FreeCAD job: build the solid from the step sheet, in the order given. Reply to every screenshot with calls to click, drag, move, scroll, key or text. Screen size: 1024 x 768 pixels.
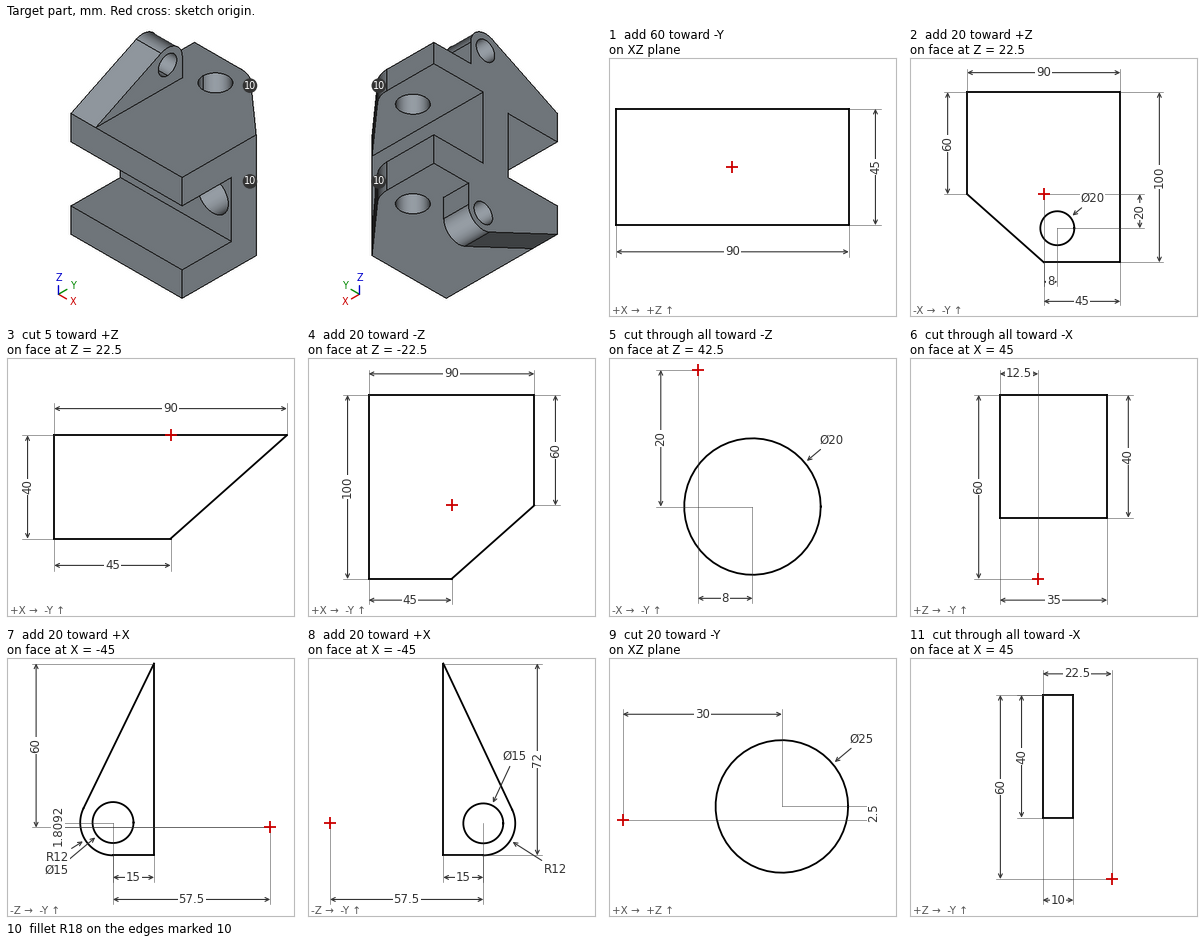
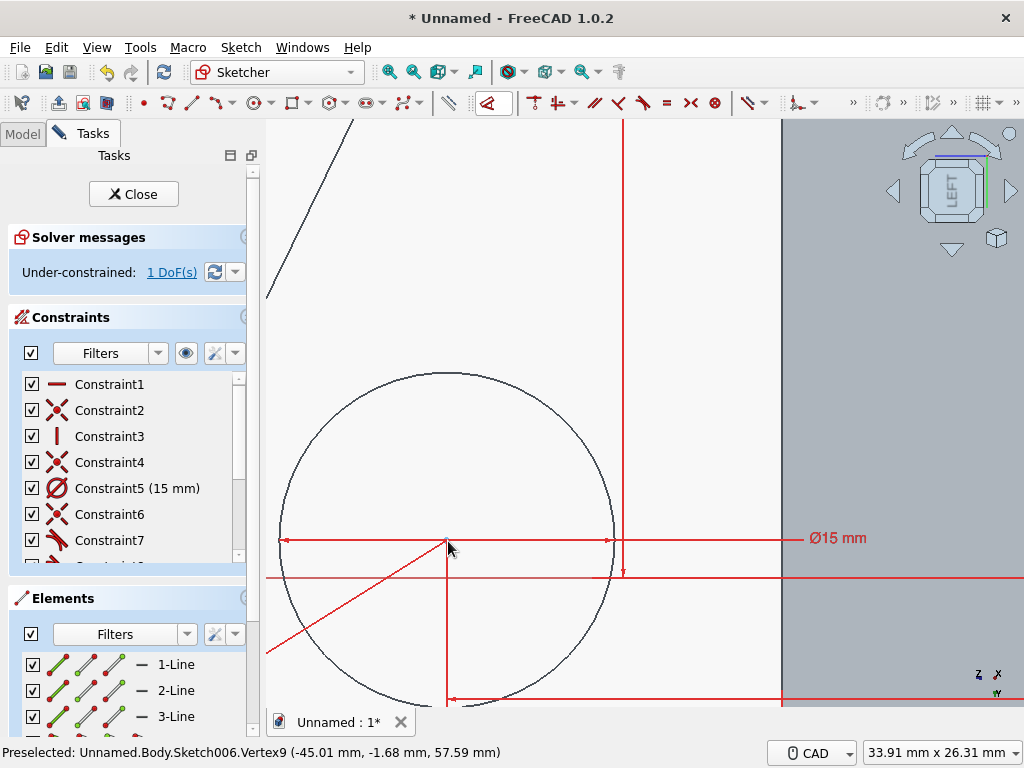
click(447, 540)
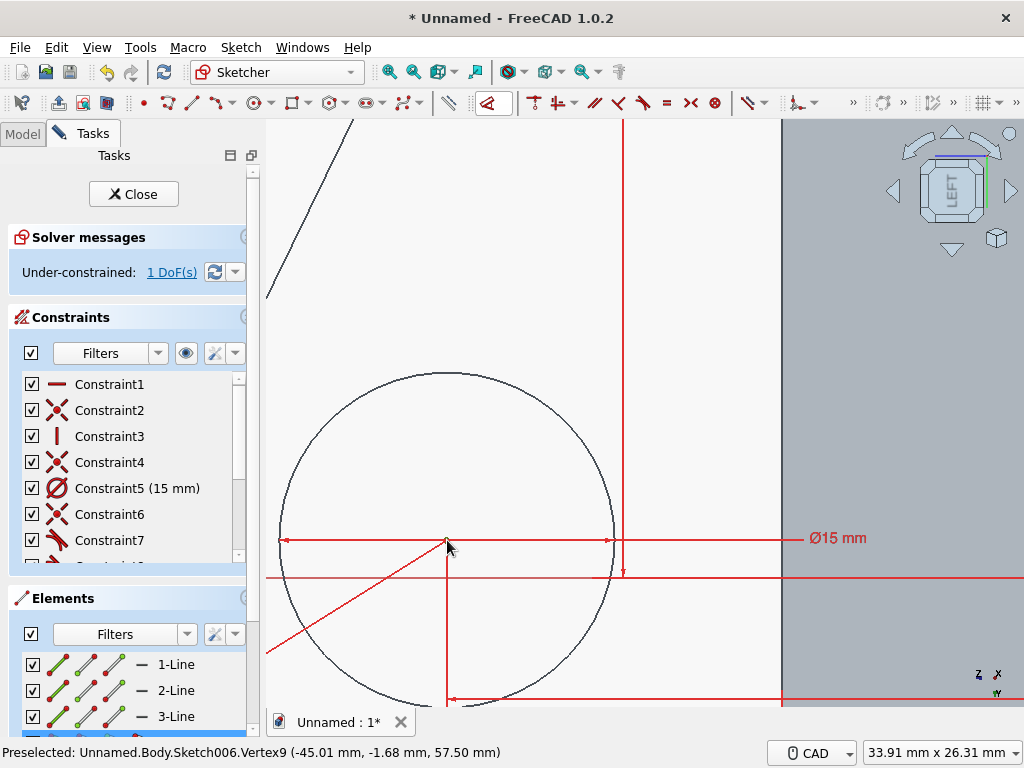
key(i)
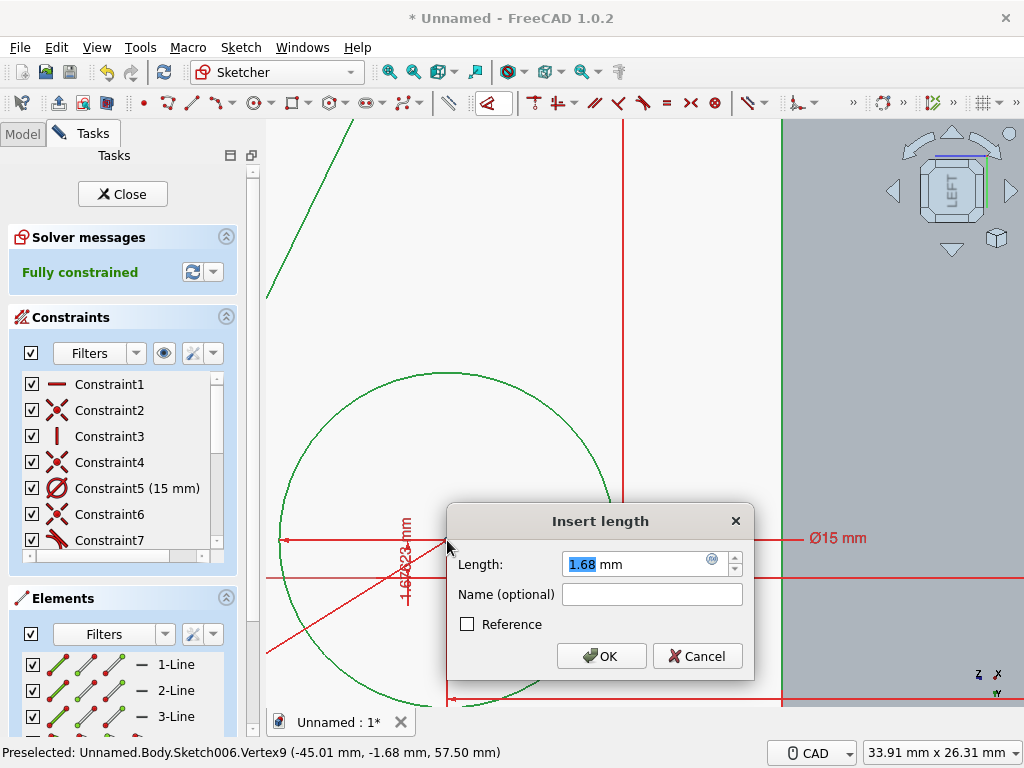
text(1.8092)
key(Return)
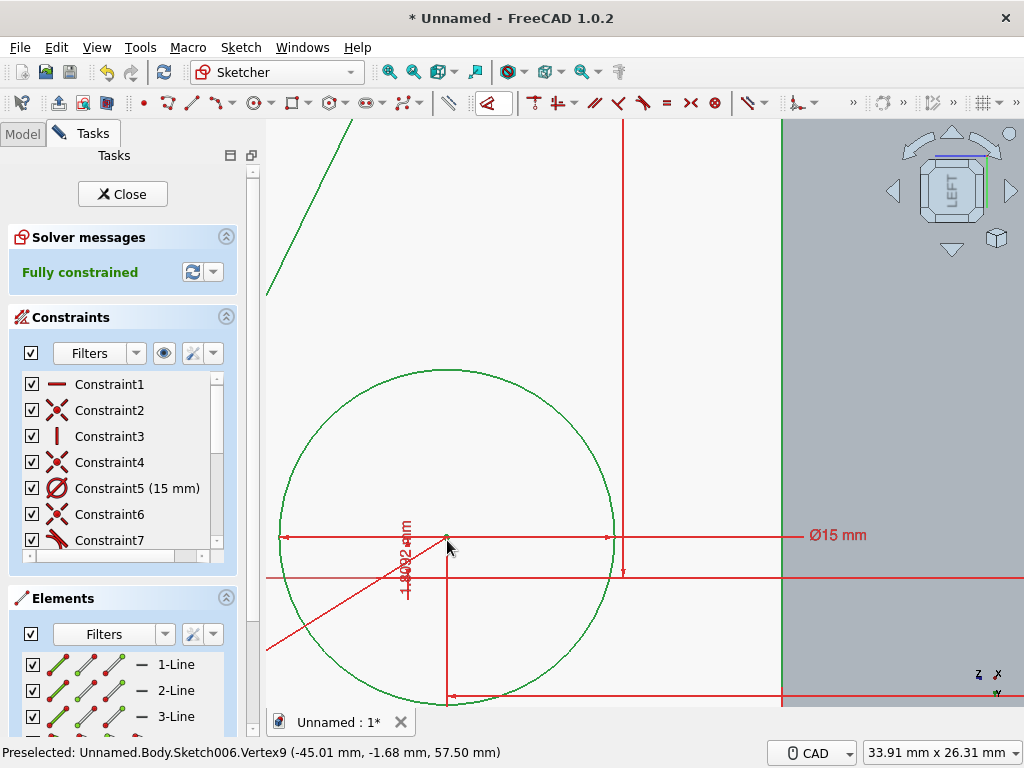
click(123, 194)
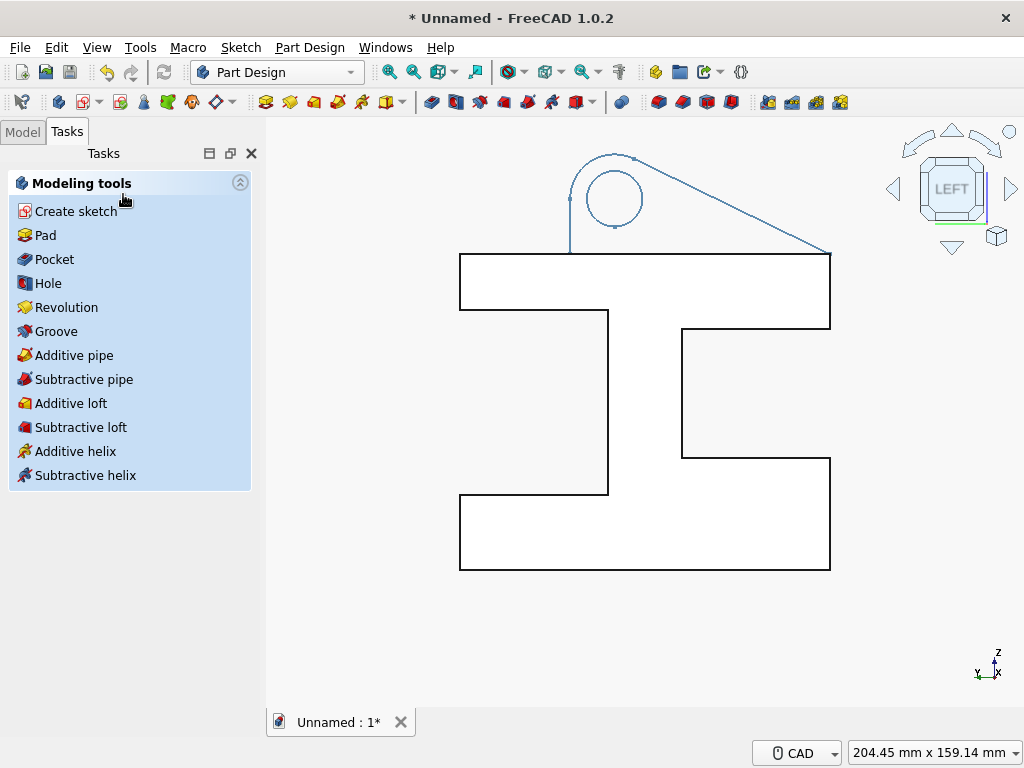
click(266, 102)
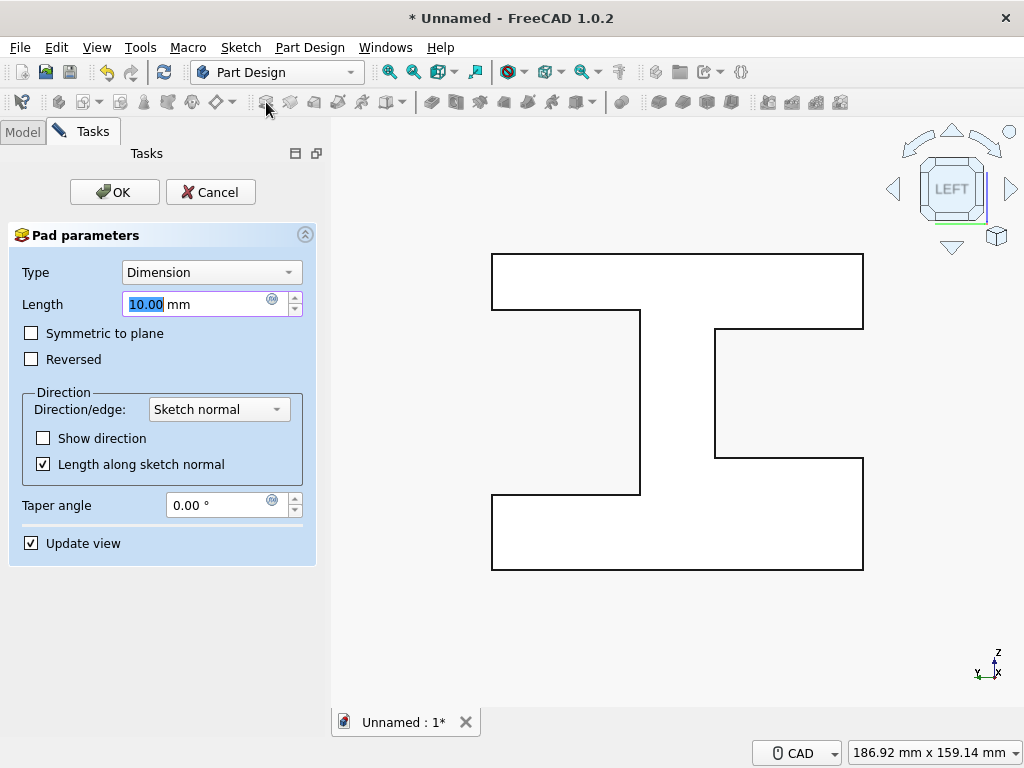
text(20)
key(Tab)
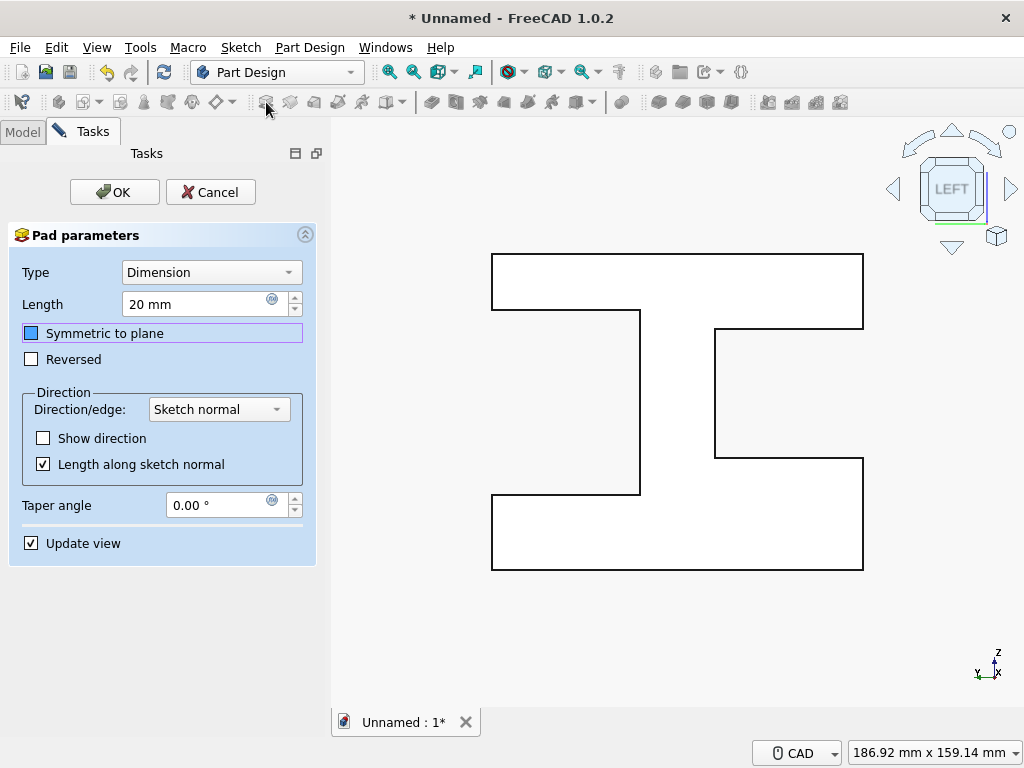
click(30, 359)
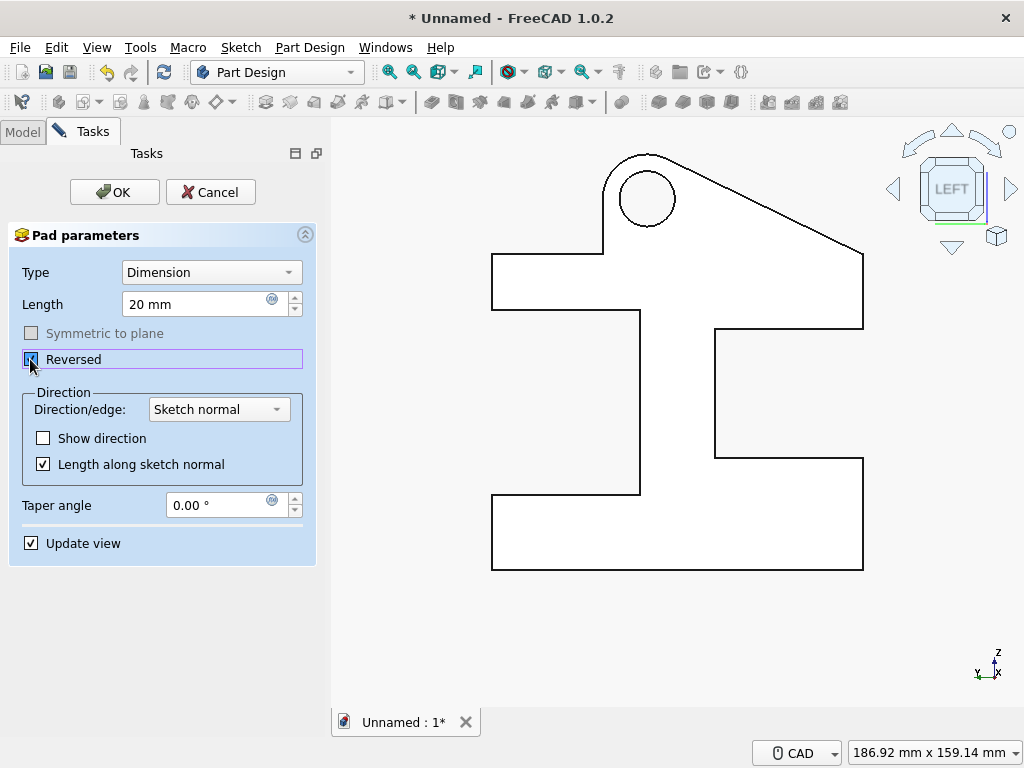
click(115, 192)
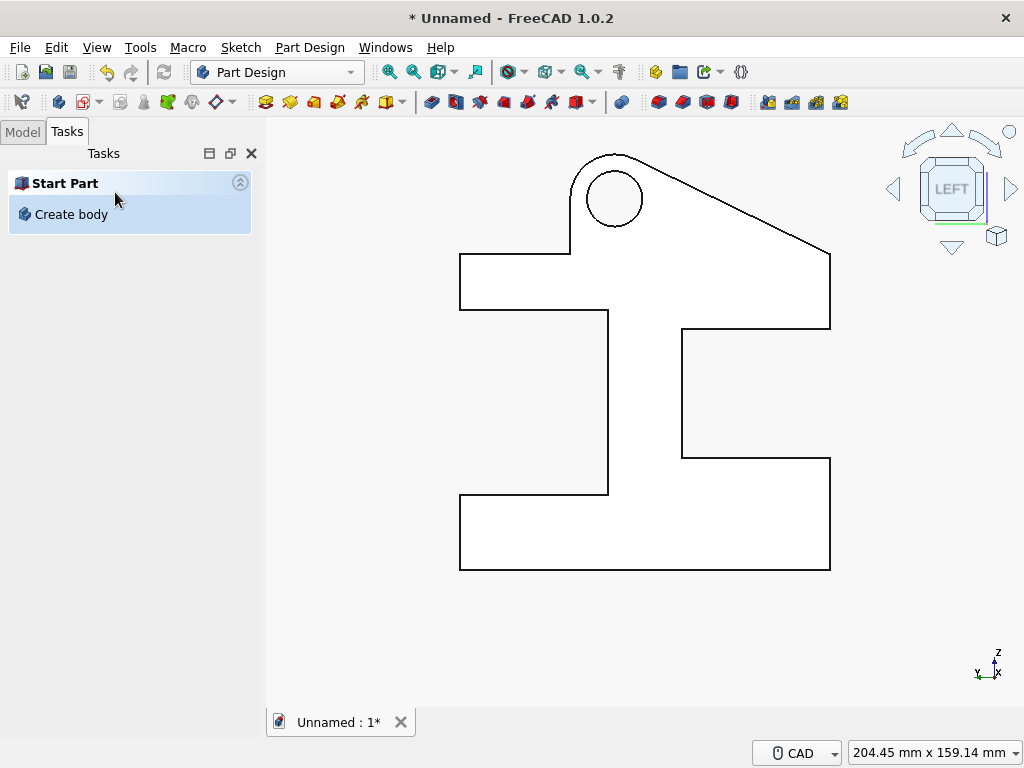
click(698, 242)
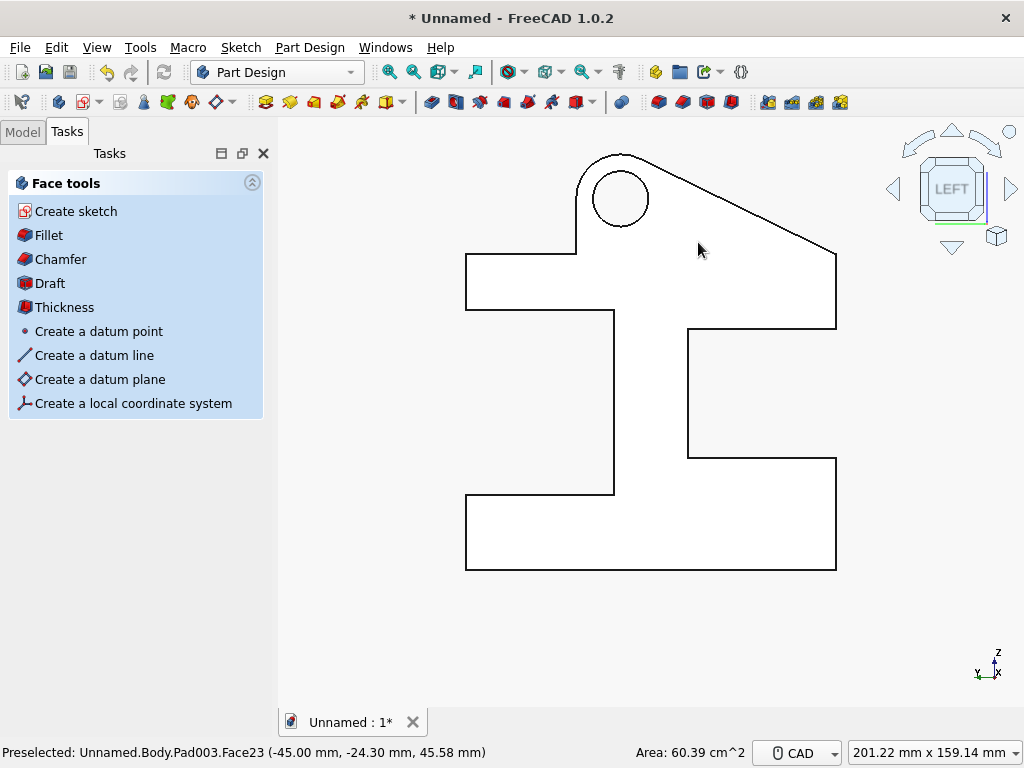
click(84, 102)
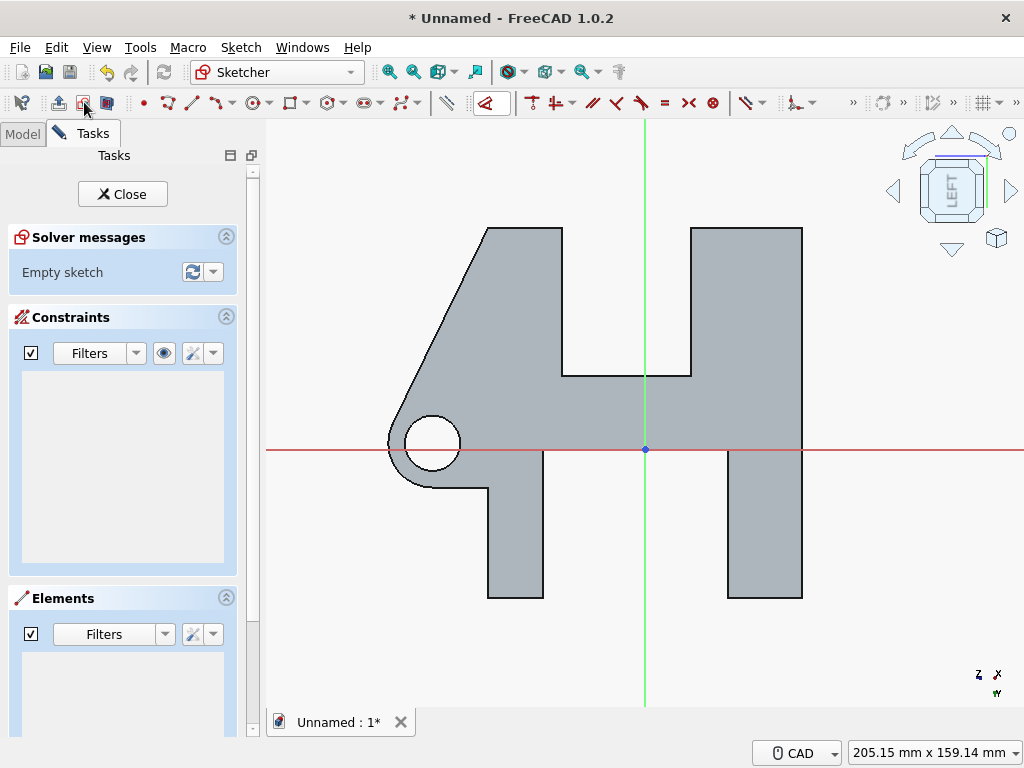
scroll(294, 647, down, 1)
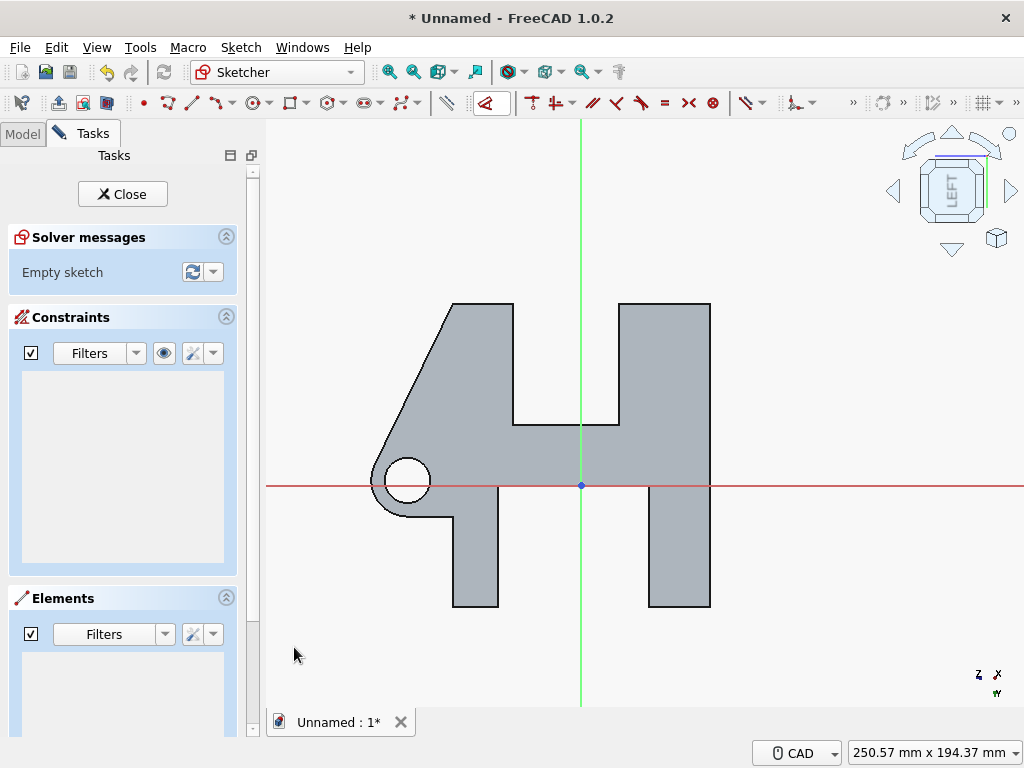
scroll(816, 414, up, 3)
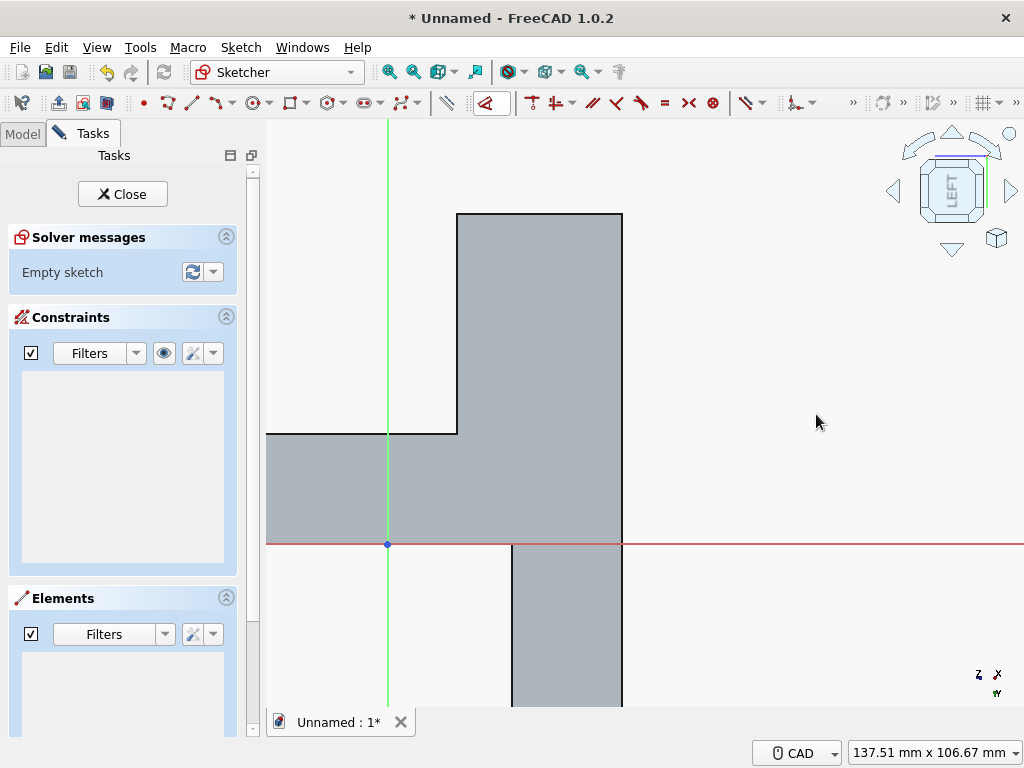
key(g)
key(m)